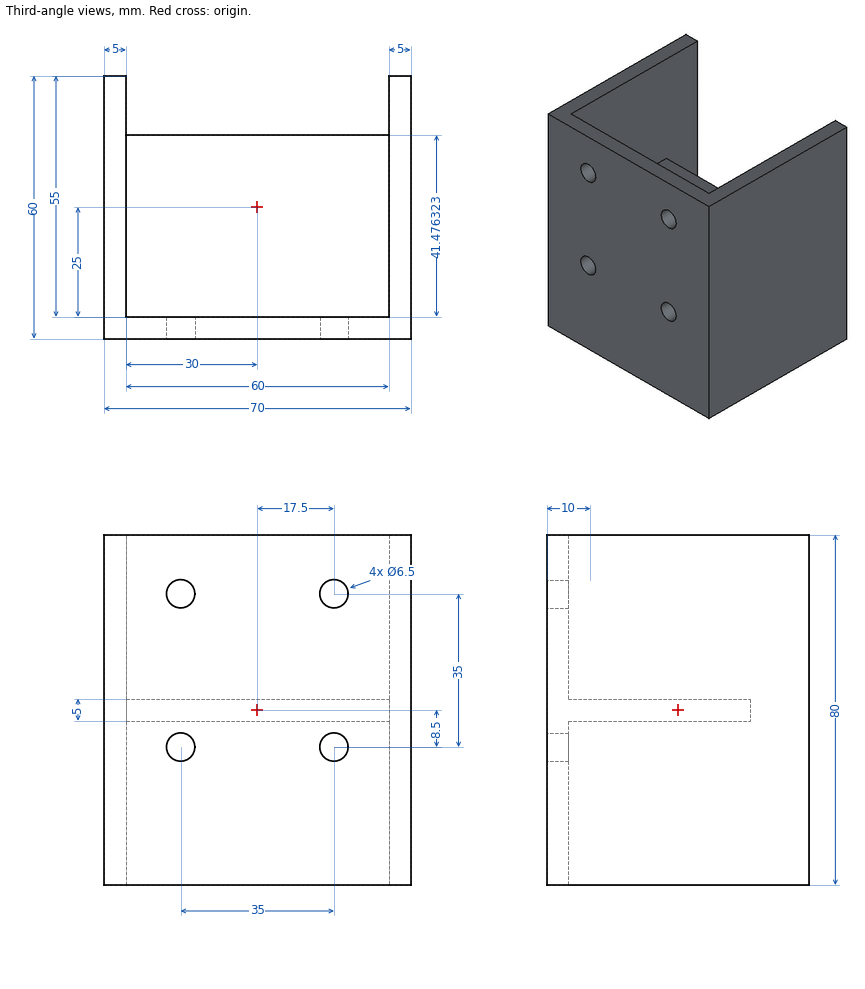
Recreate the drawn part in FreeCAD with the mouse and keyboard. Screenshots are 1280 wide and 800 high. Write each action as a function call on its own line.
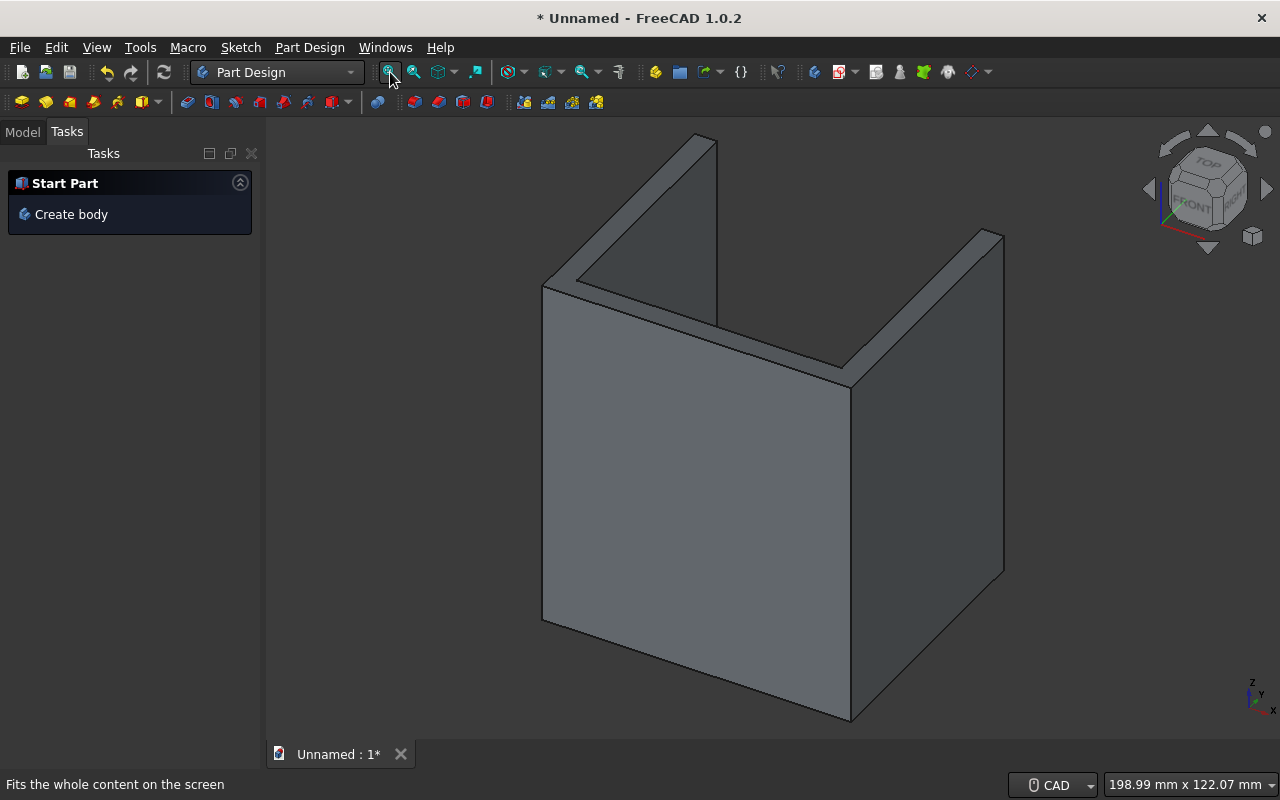
click(840, 72)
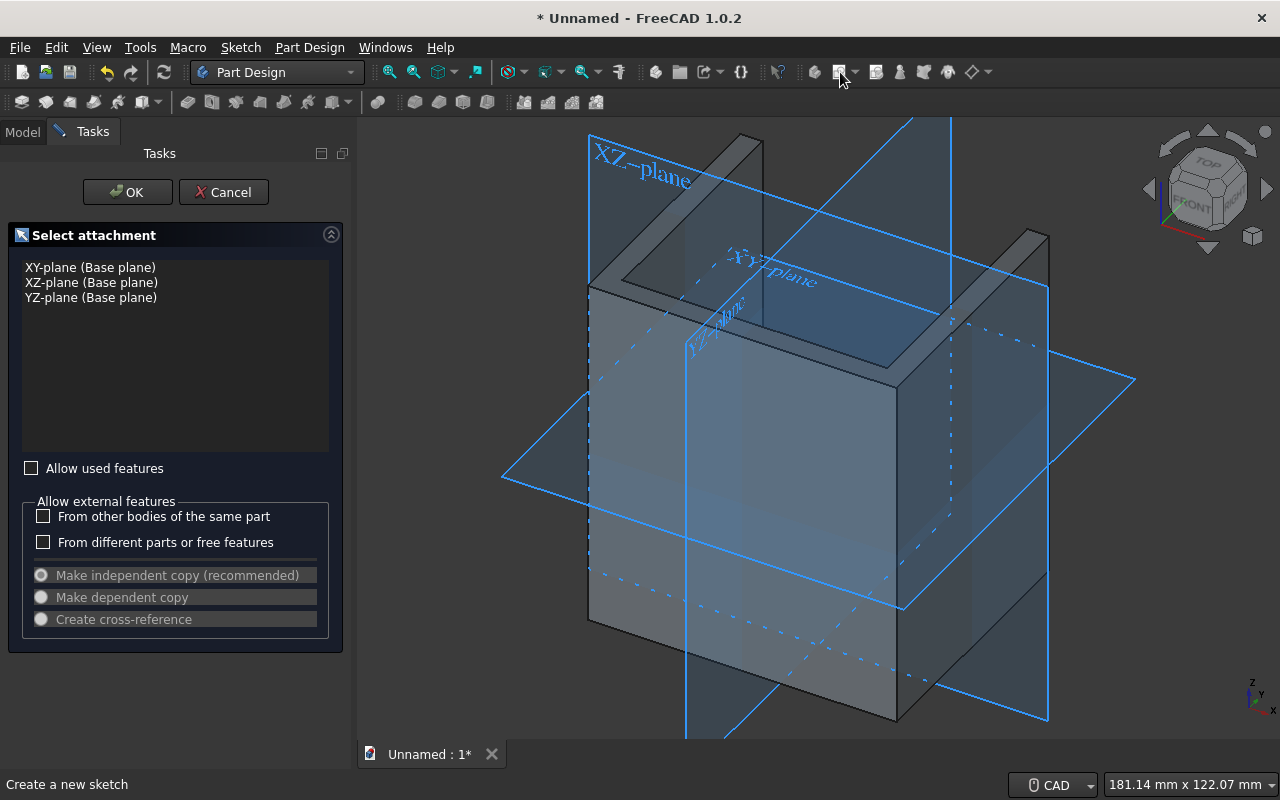
click(82, 268)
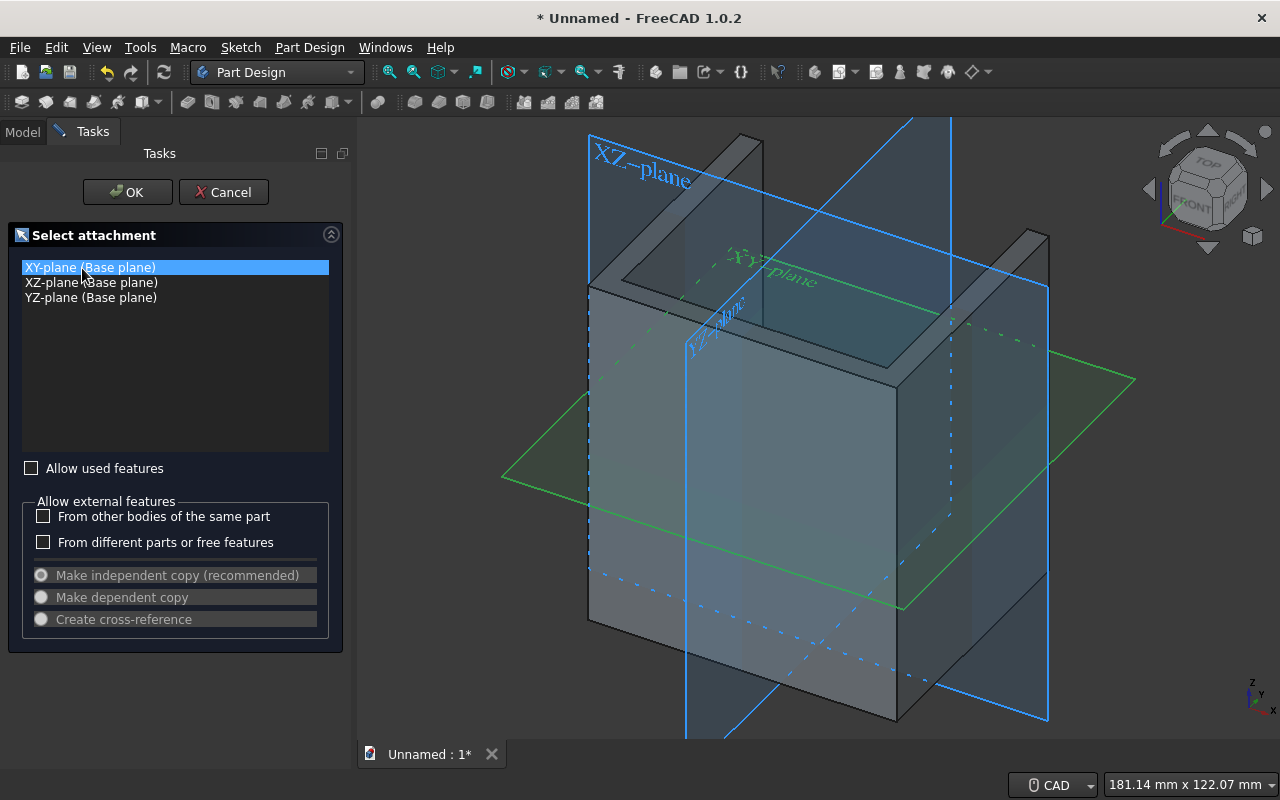
click(128, 192)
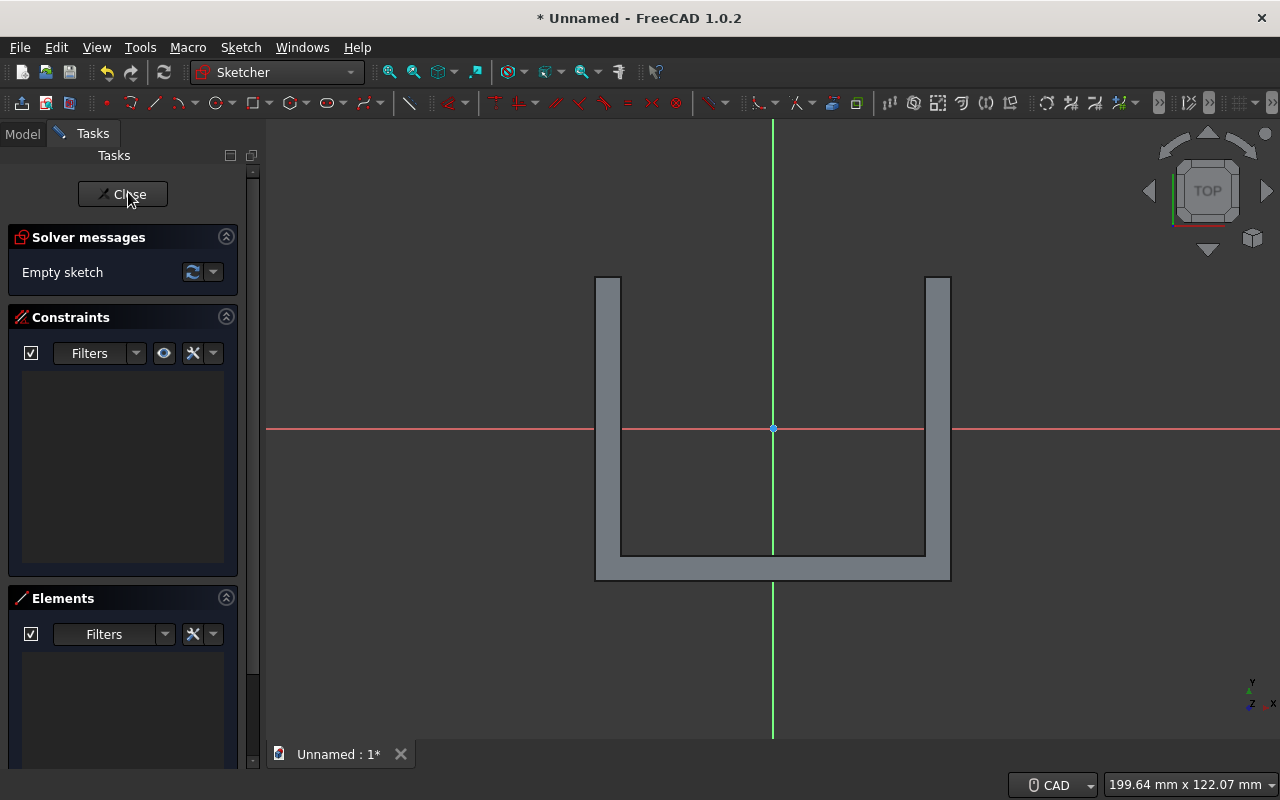
click(70, 104)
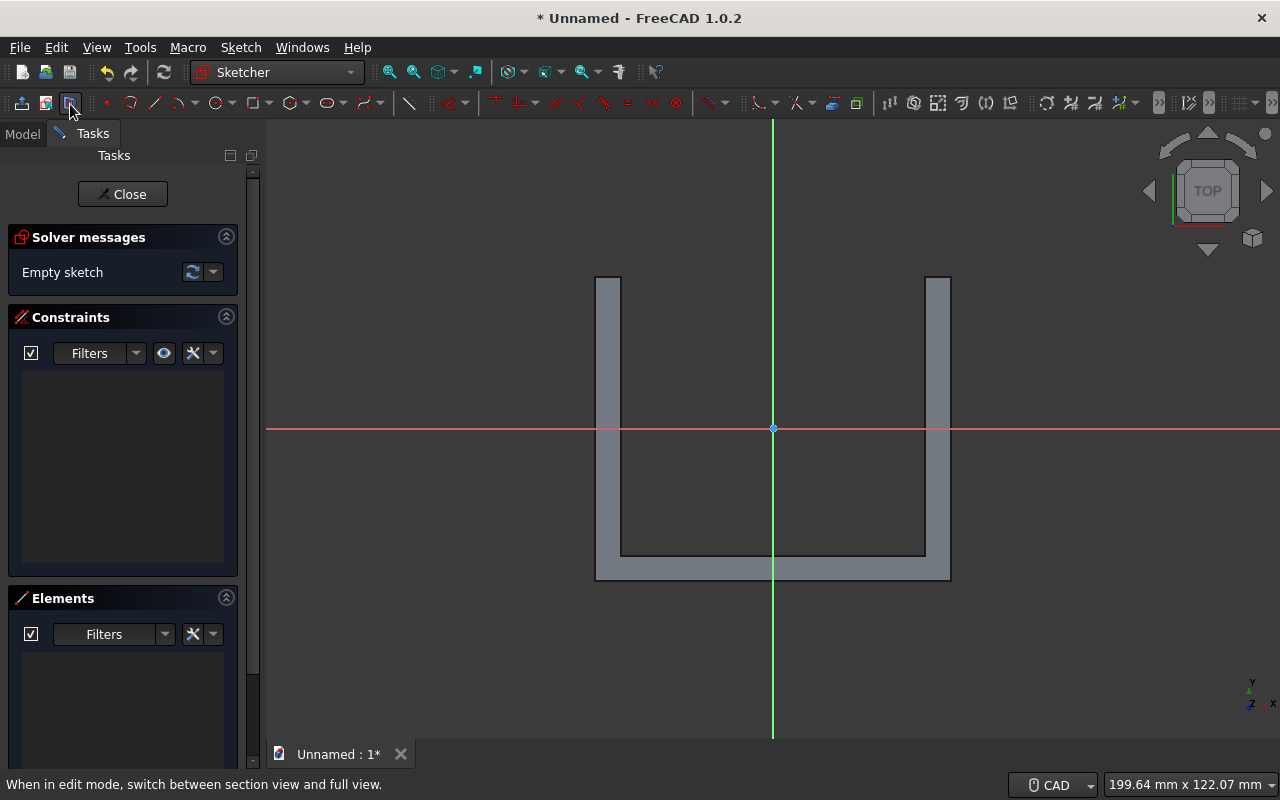
scroll(856, 477, up, 3)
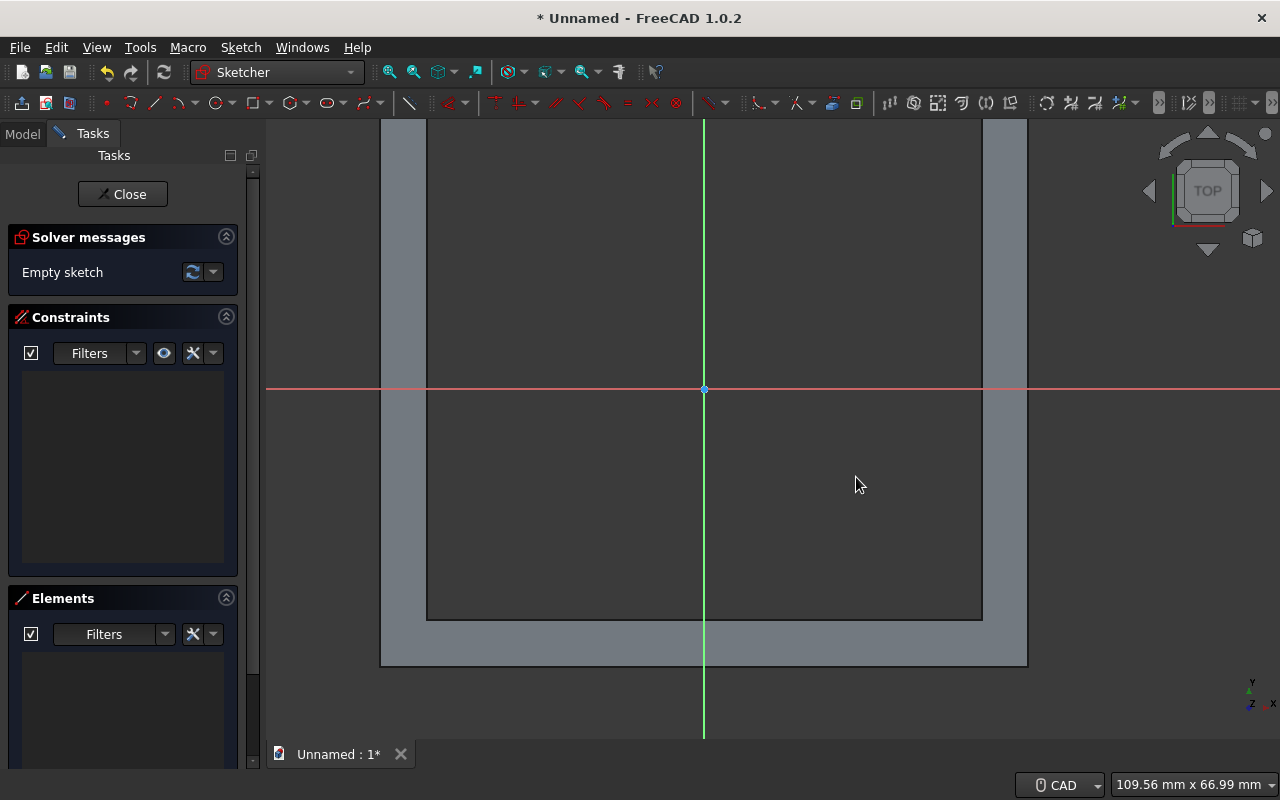
key(g)
key(r)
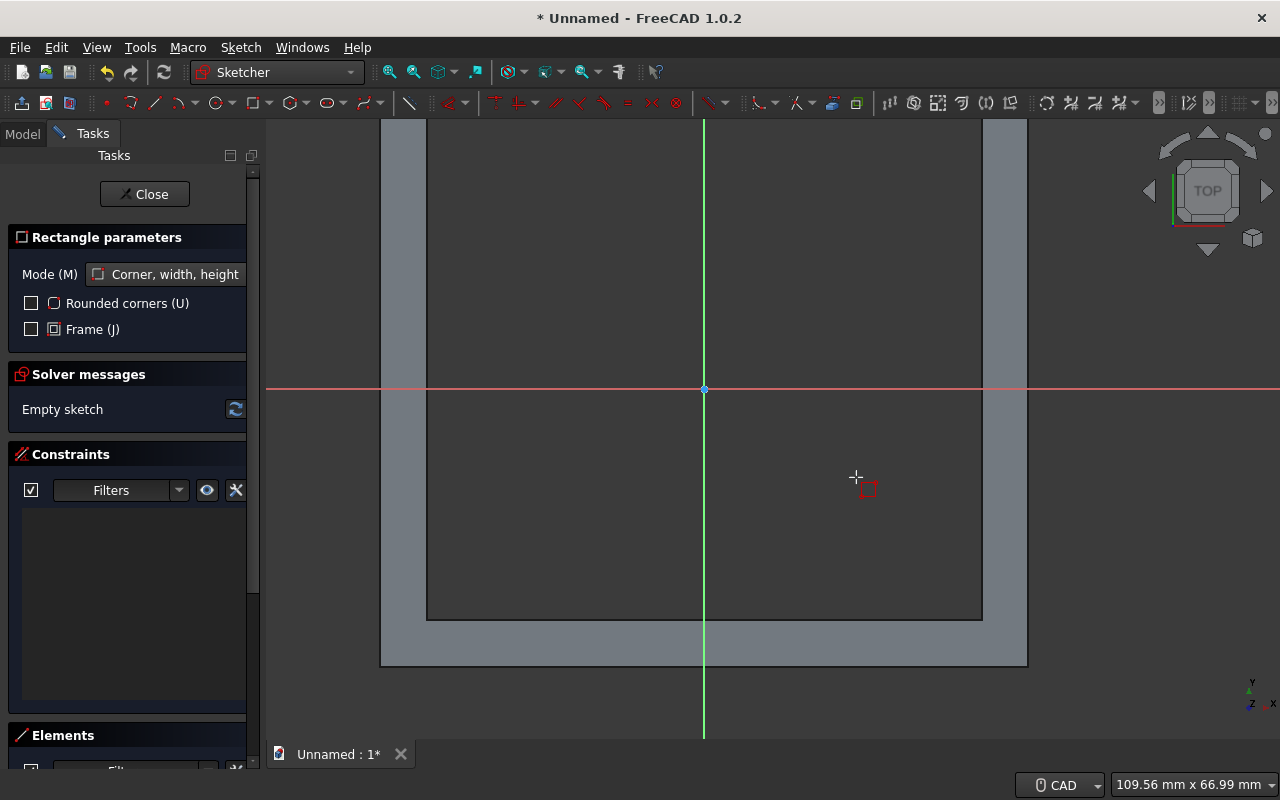
click(427, 237)
move(982, 620)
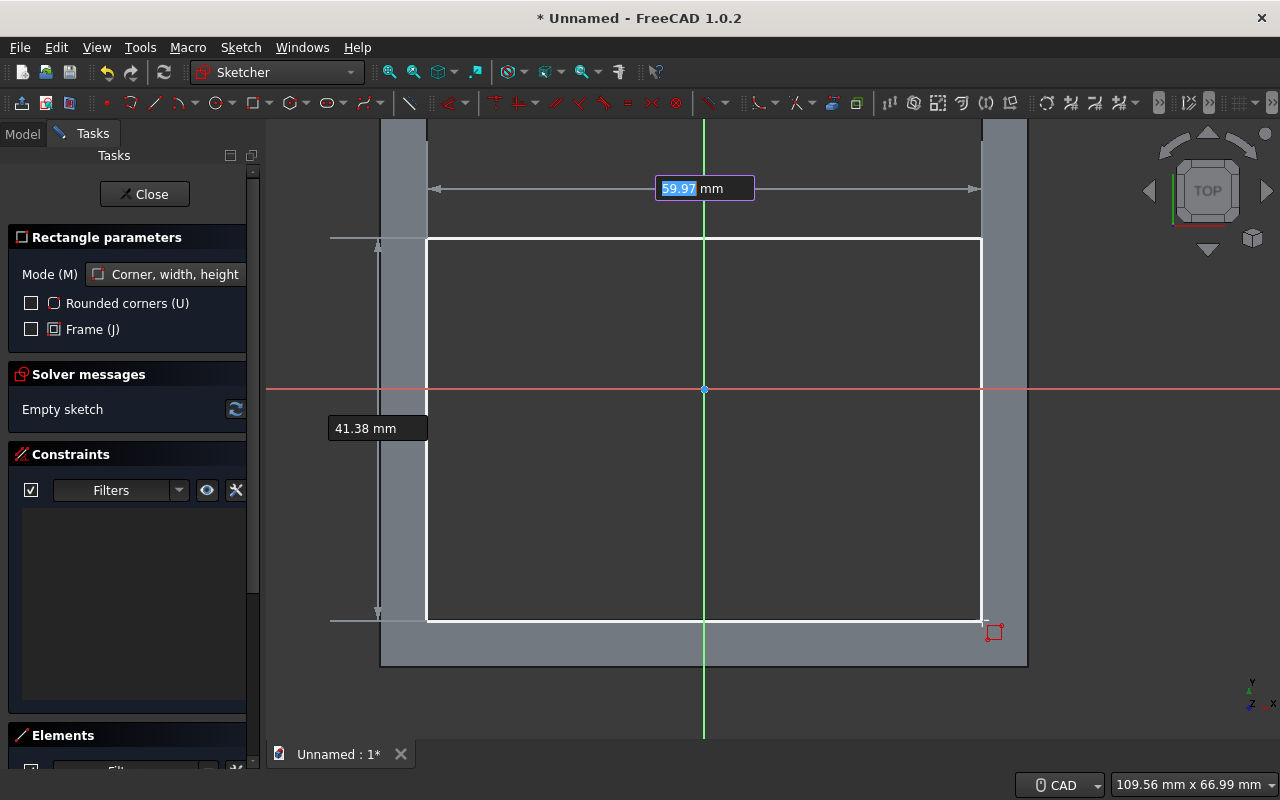
text(60)
key(Tab)
text(41.476323)
key(Return)
key(Escape)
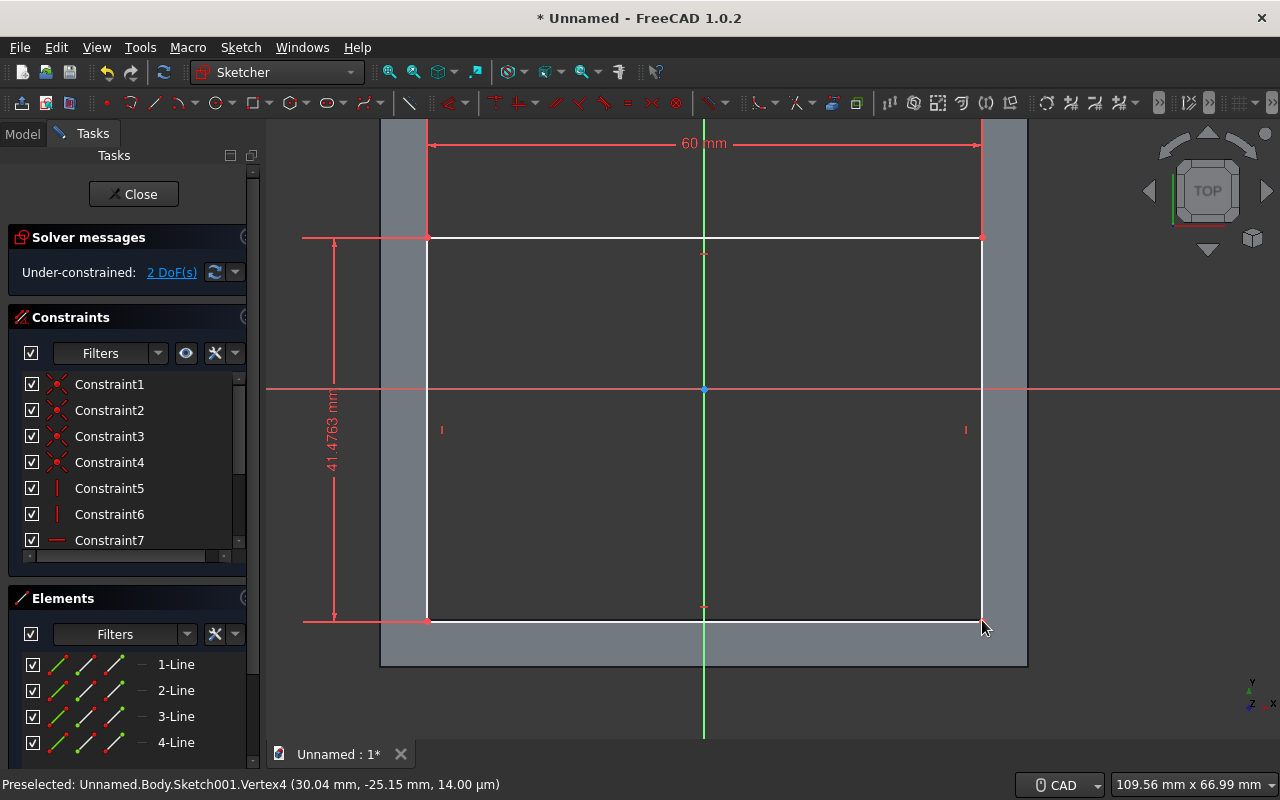
click(427, 238)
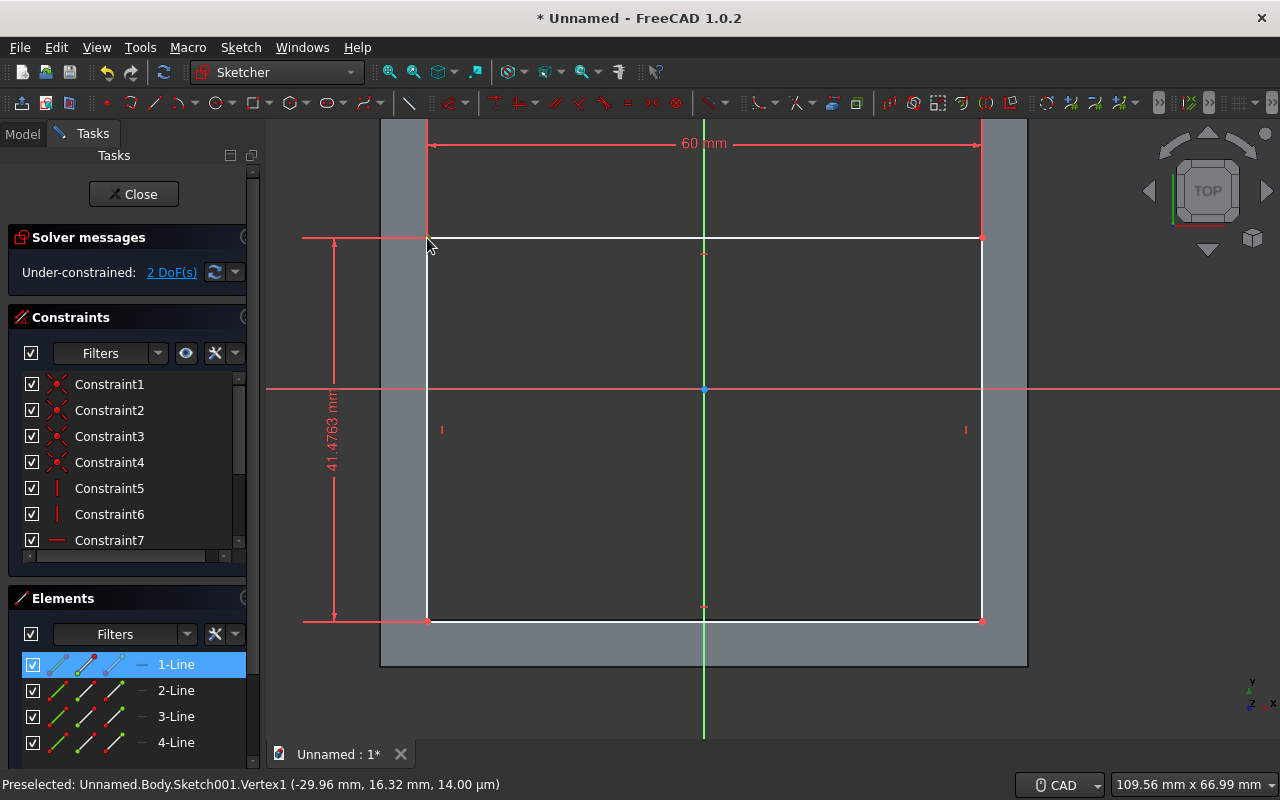
key(l)